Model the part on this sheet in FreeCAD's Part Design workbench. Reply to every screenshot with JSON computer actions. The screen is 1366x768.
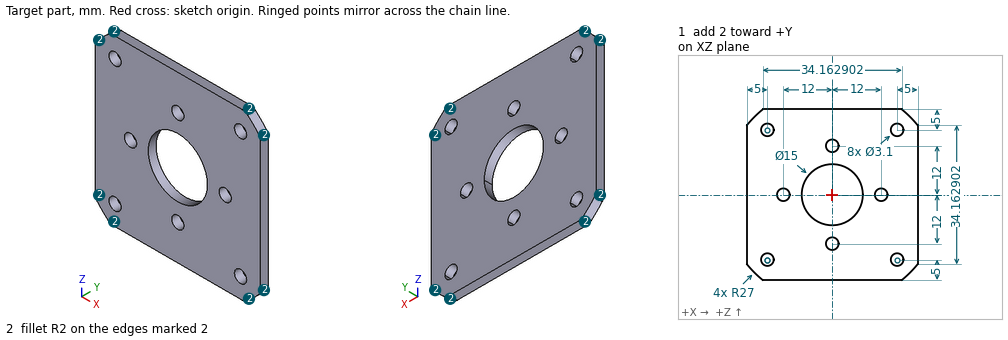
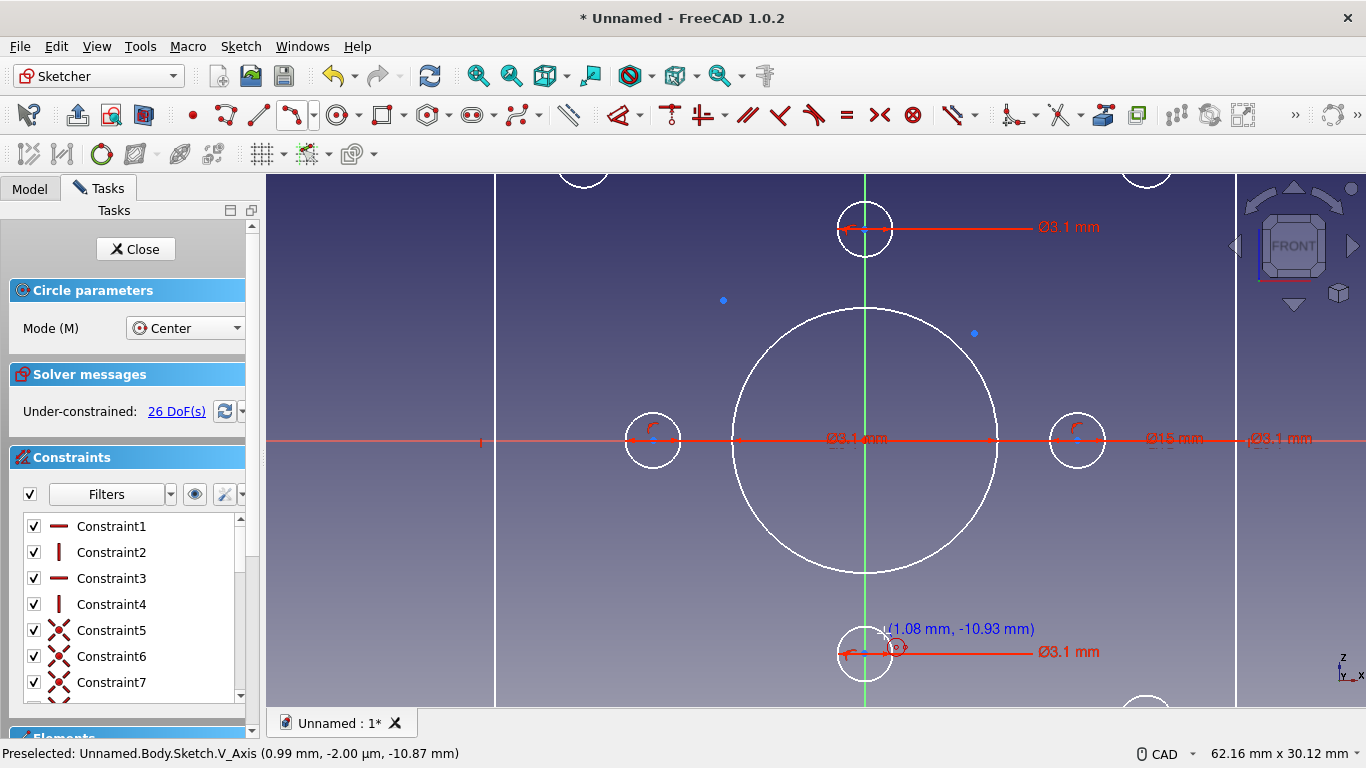
{"action": "scroll", "coordinate": [652, 440], "scroll_direction": "down", "scroll_amount": 4}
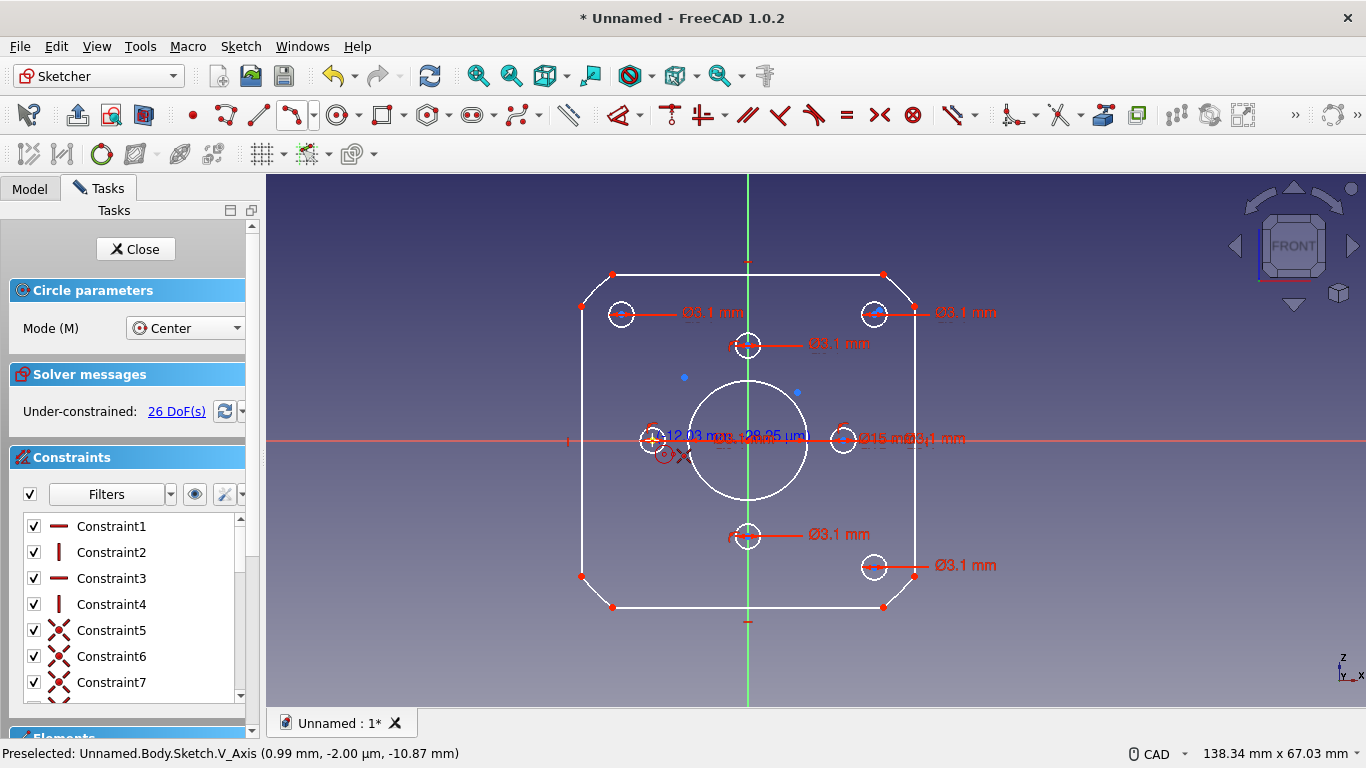
{"action": "scroll", "coordinate": [621, 567], "scroll_direction": "up", "scroll_amount": 4}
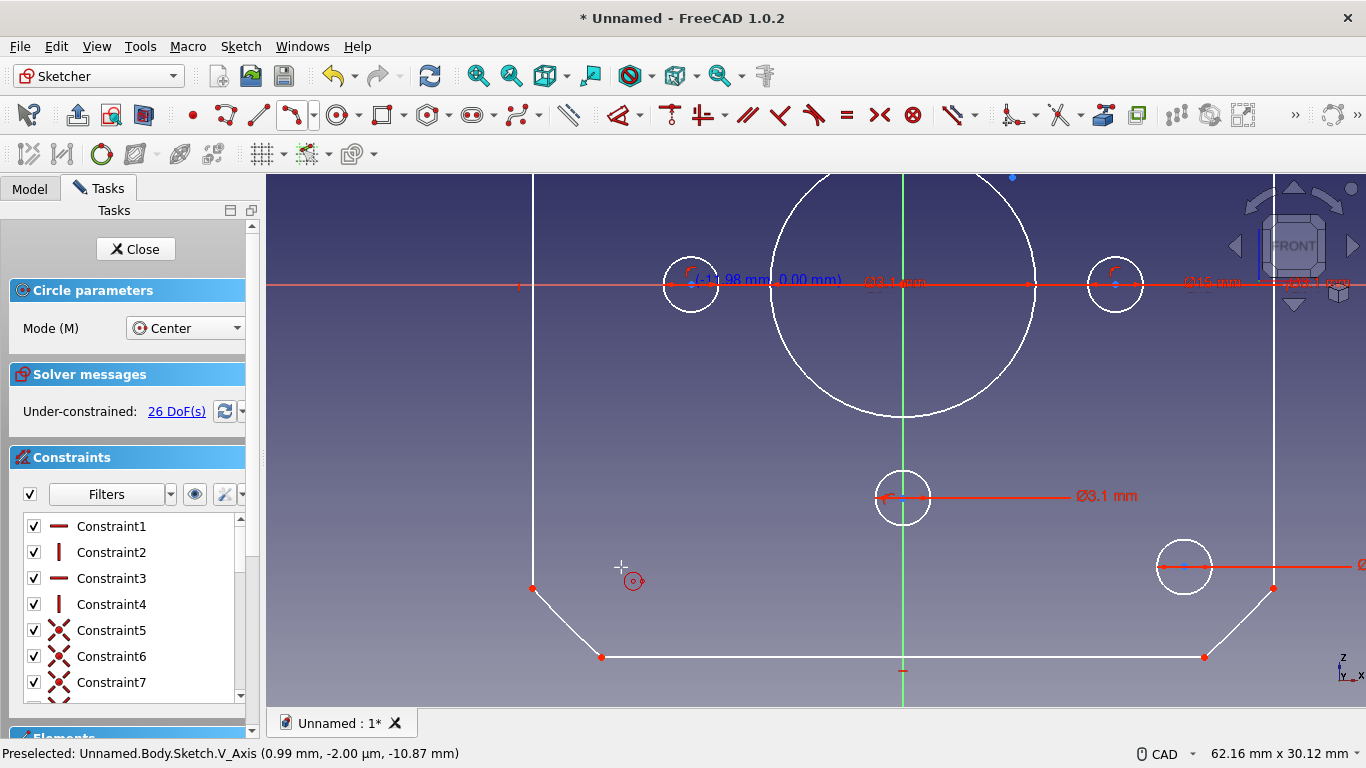
{"action": "left_click", "coordinate": [621, 566]}
{"action": "mouse_move", "coordinate": [641, 547]}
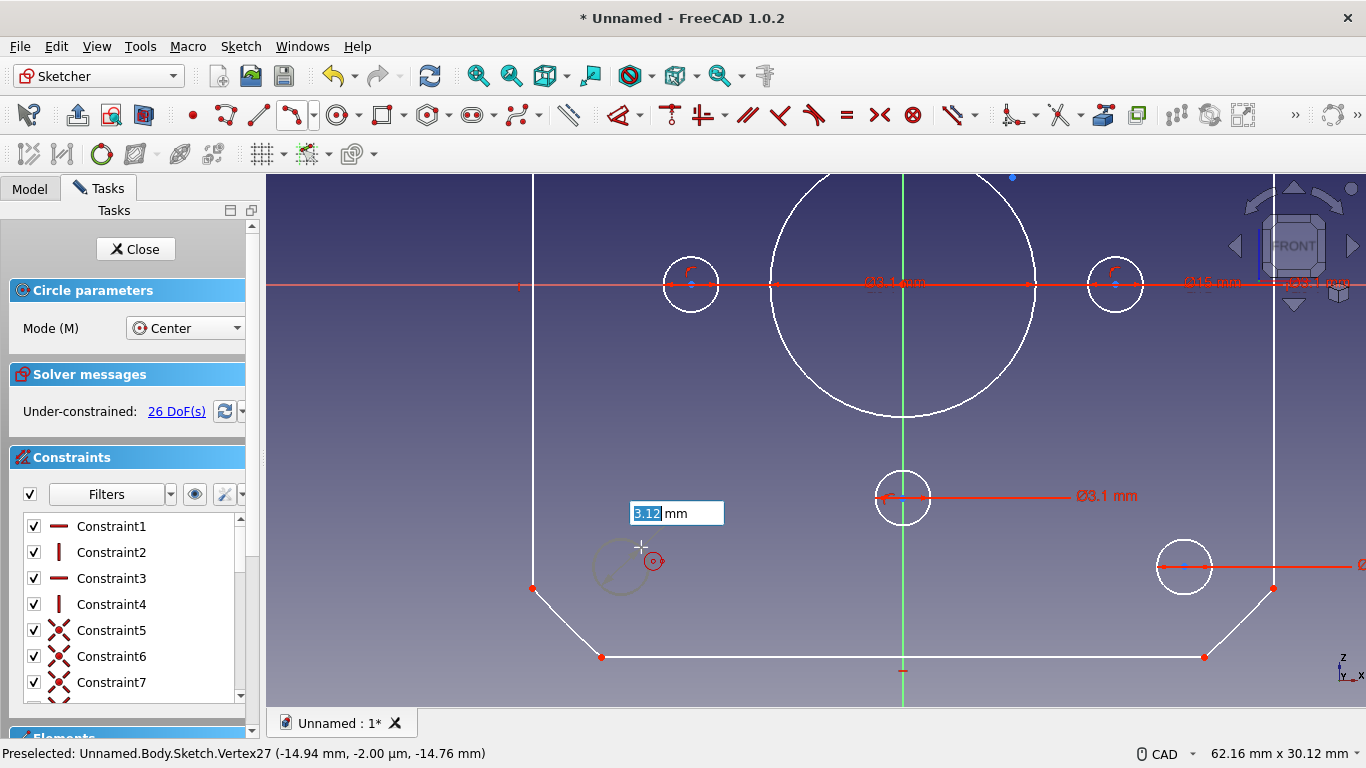
{"action": "type", "text": "3.1"}
{"action": "key", "text": "Return"}
{"action": "key", "text": "Escape"}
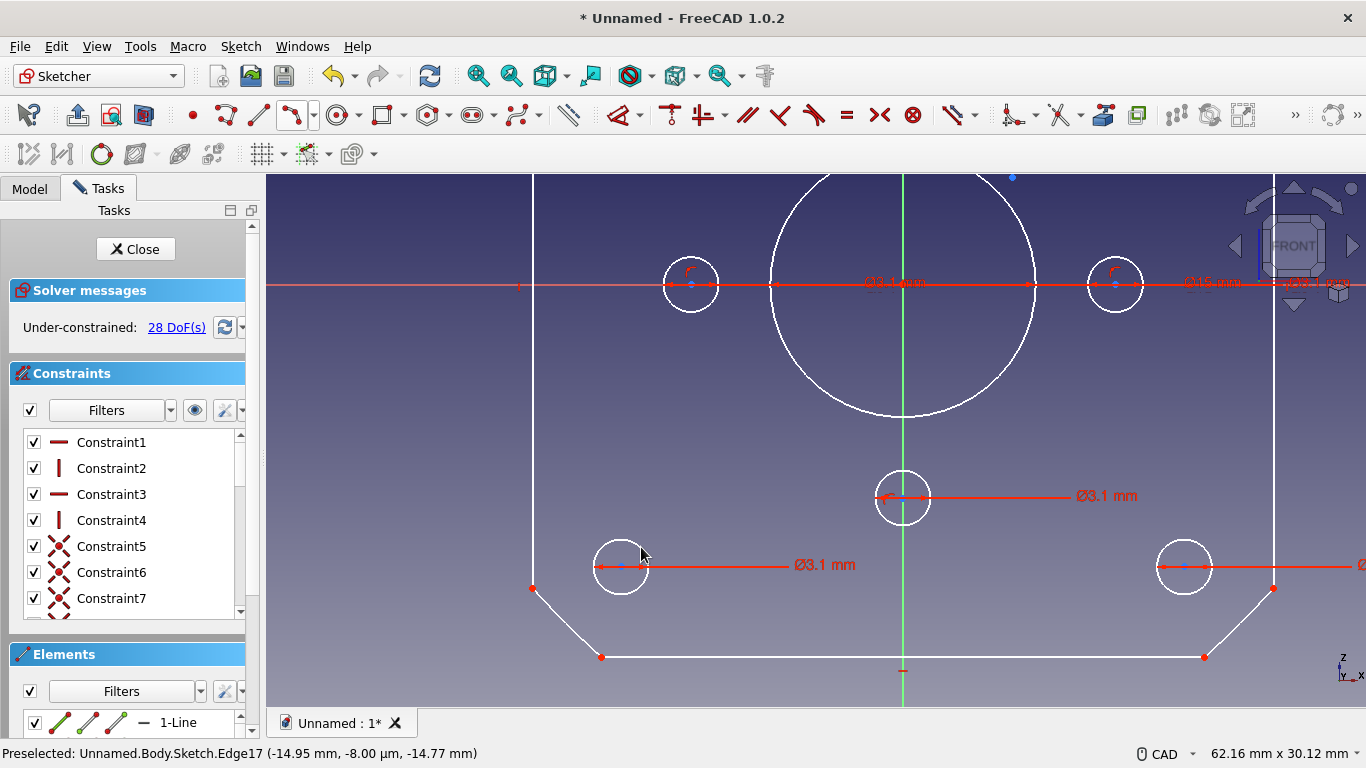
{"action": "left_click", "coordinate": [809, 379]}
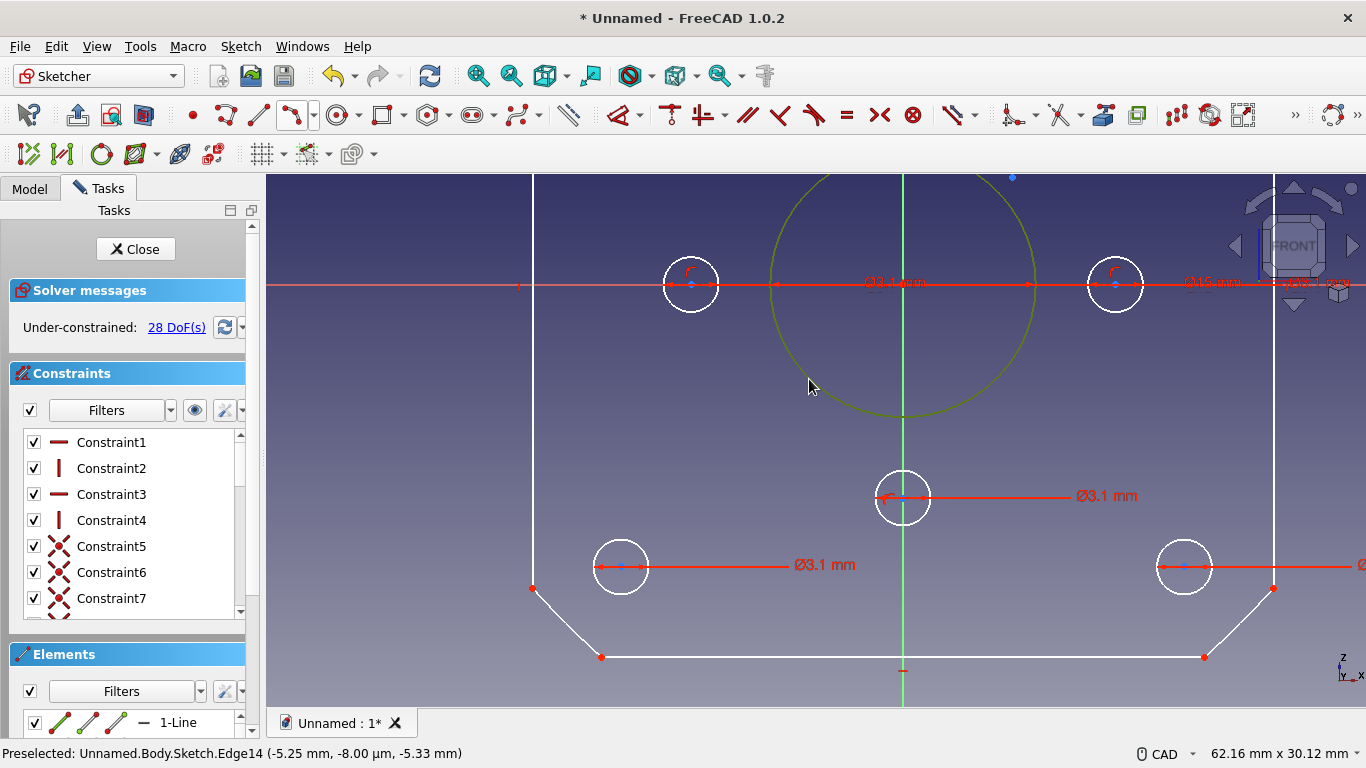
{"action": "scroll", "coordinate": [621, 568], "scroll_direction": "down", "scroll_amount": 4}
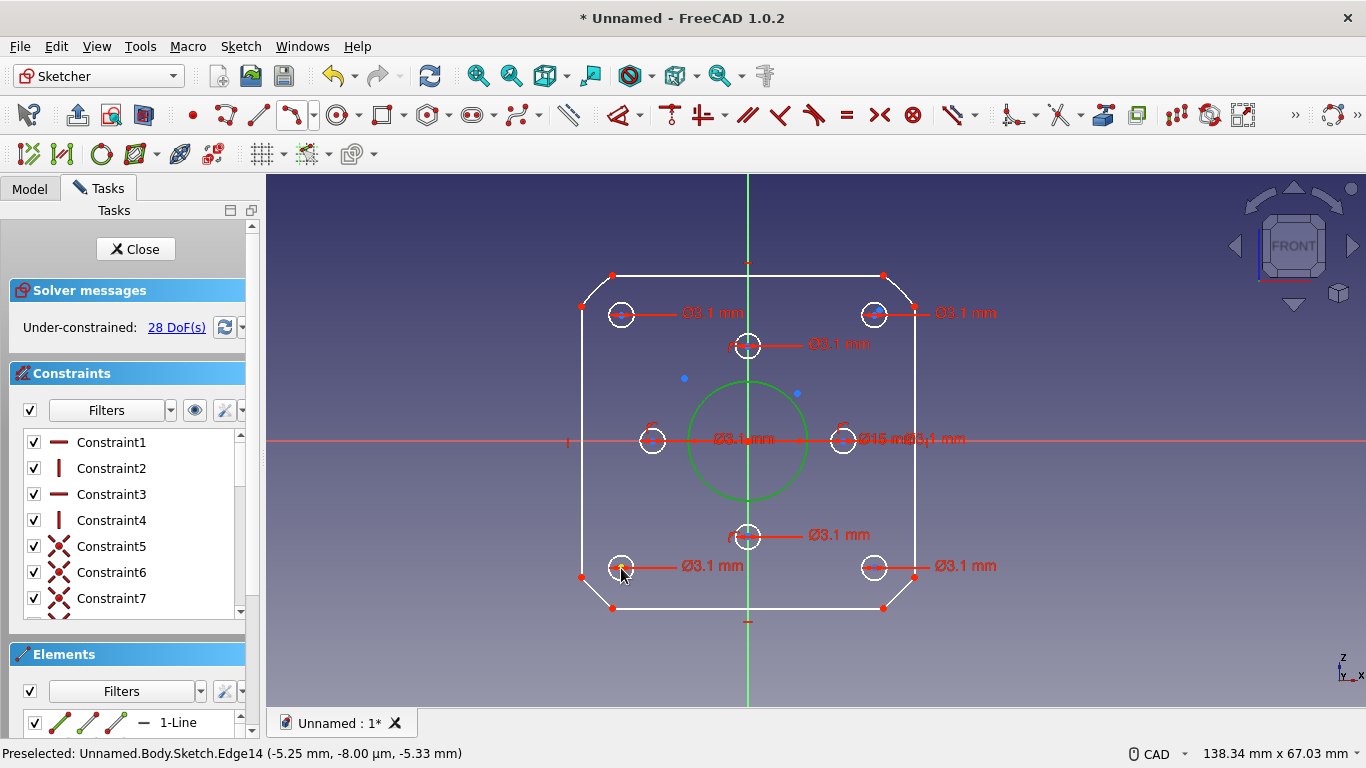
{"action": "left_click", "coordinate": [906, 296]}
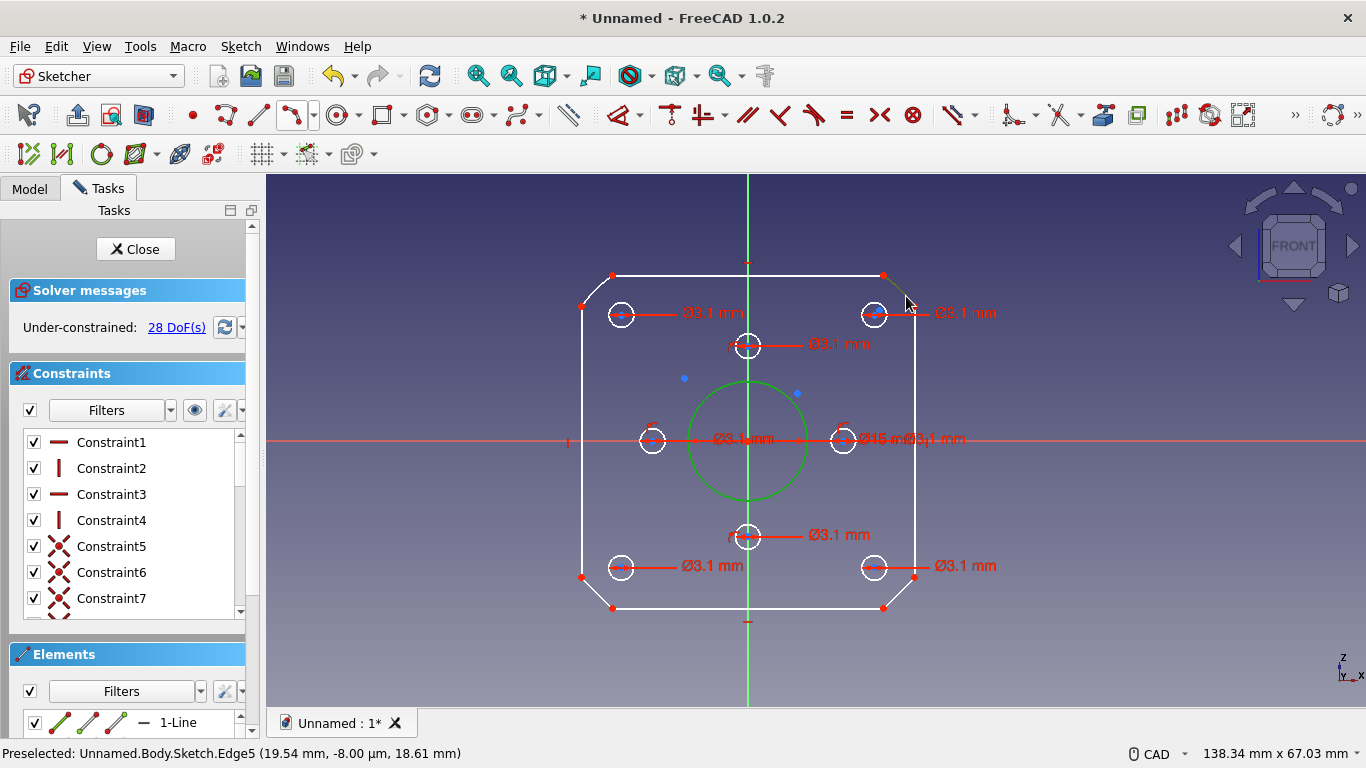
{"action": "left_click", "coordinate": [670, 116]}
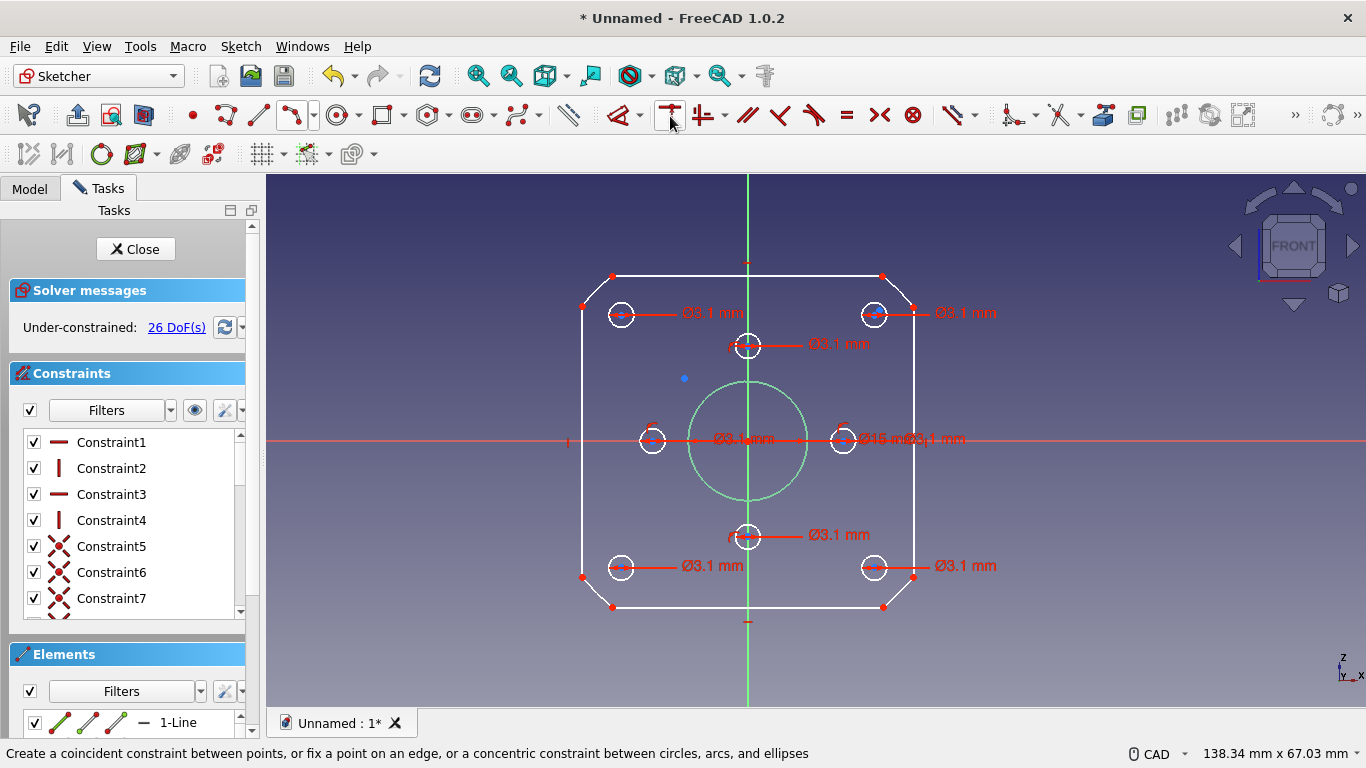
{"action": "left_click", "coordinate": [790, 399]}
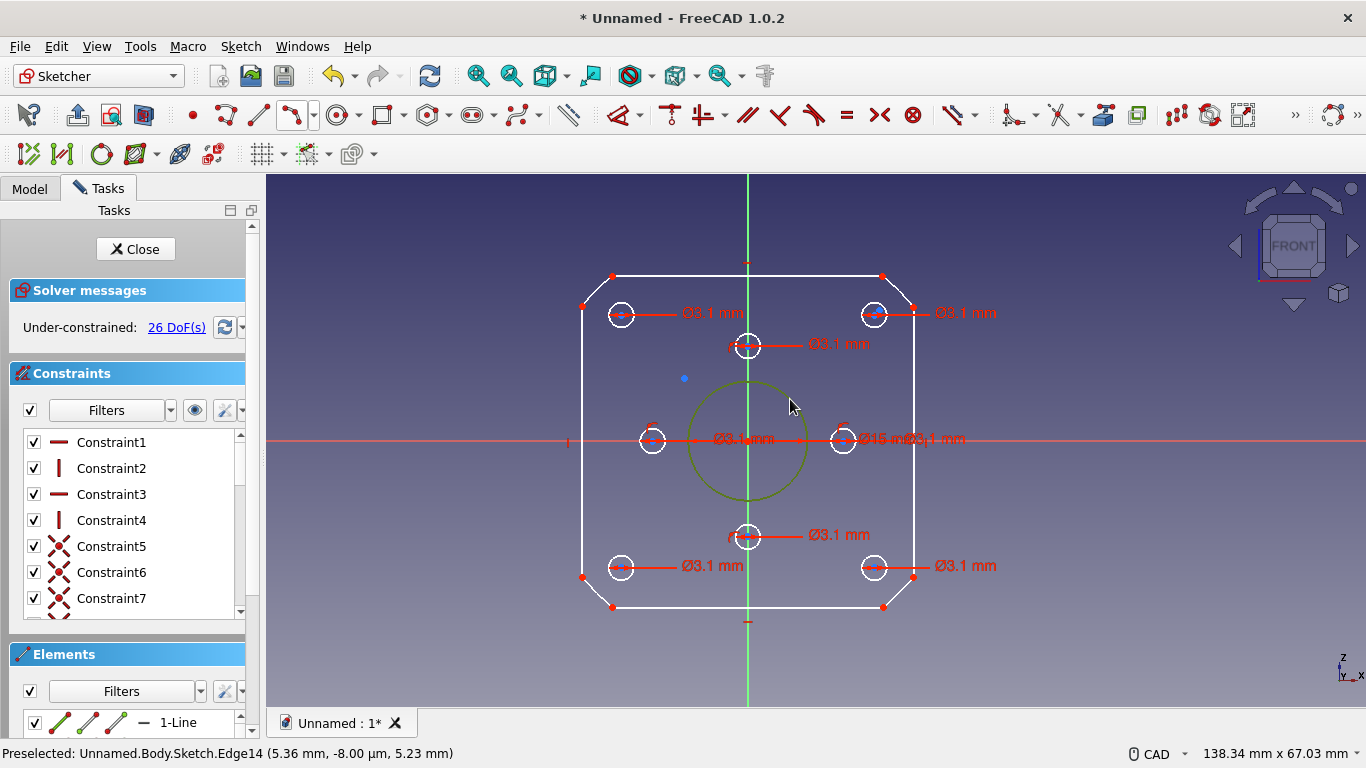
{"action": "left_click", "coordinate": [893, 599]}